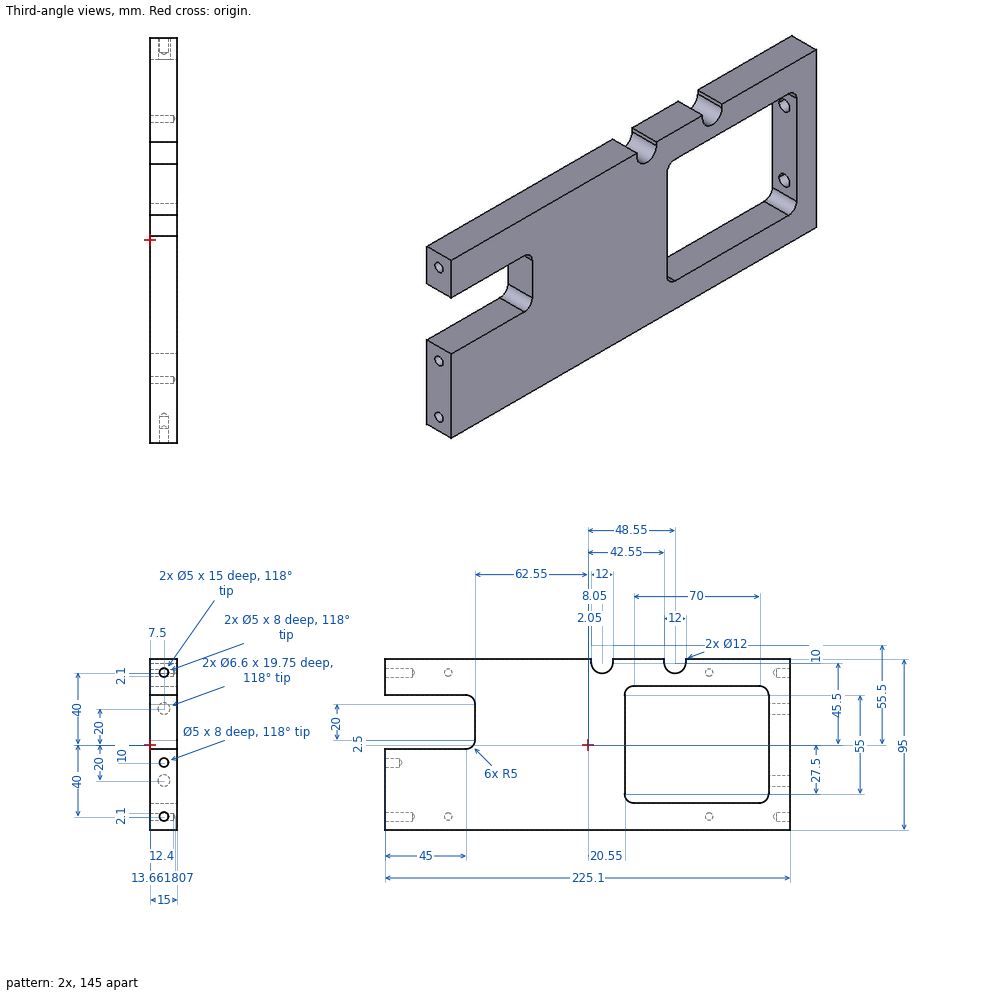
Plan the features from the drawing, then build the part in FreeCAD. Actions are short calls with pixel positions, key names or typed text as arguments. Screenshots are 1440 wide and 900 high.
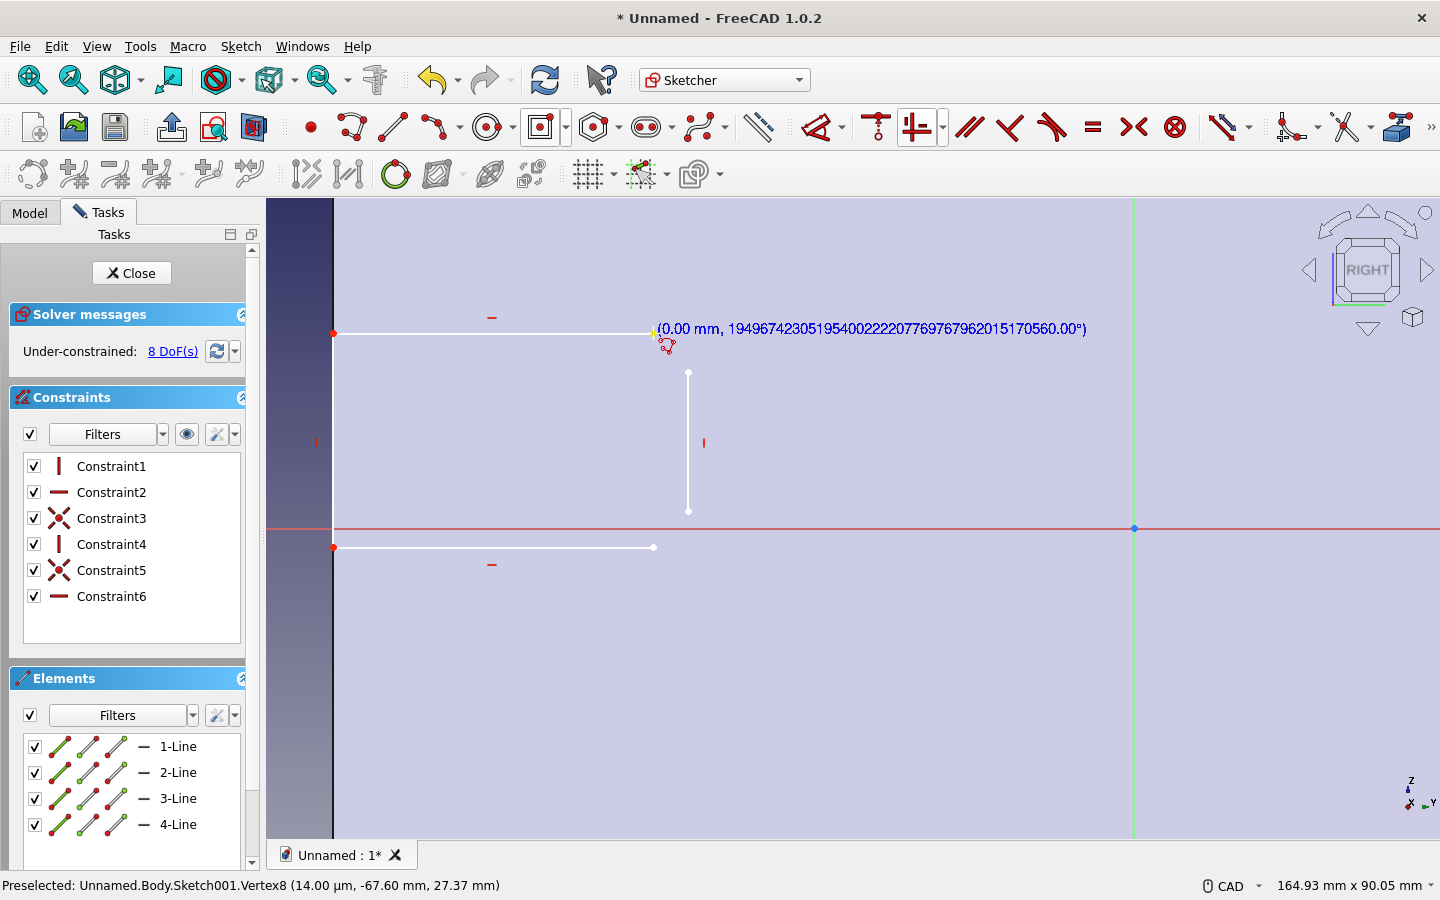
click(434, 128)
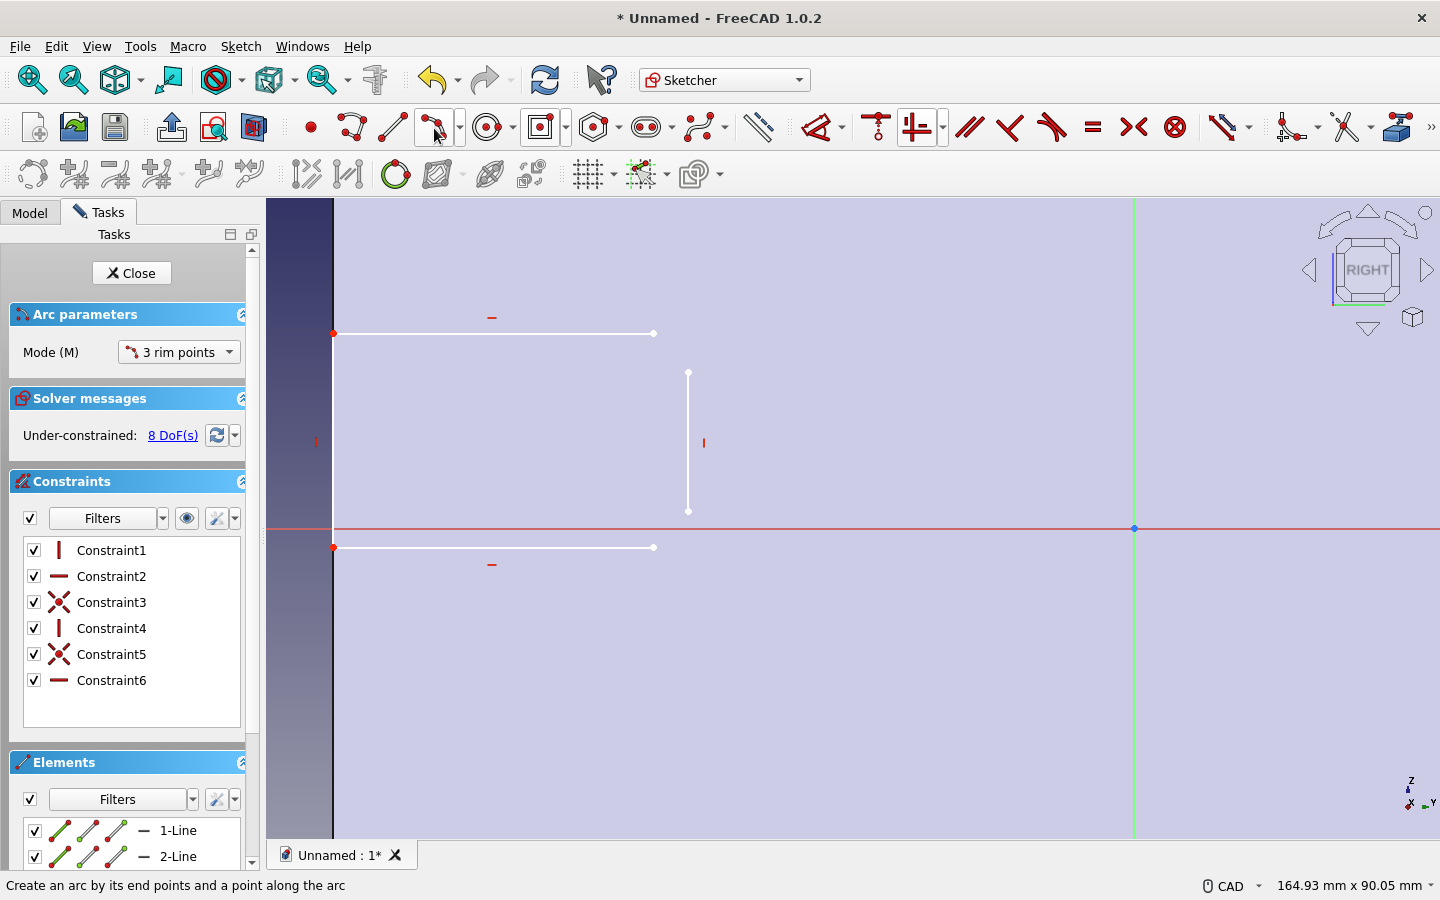
click(688, 512)
click(653, 548)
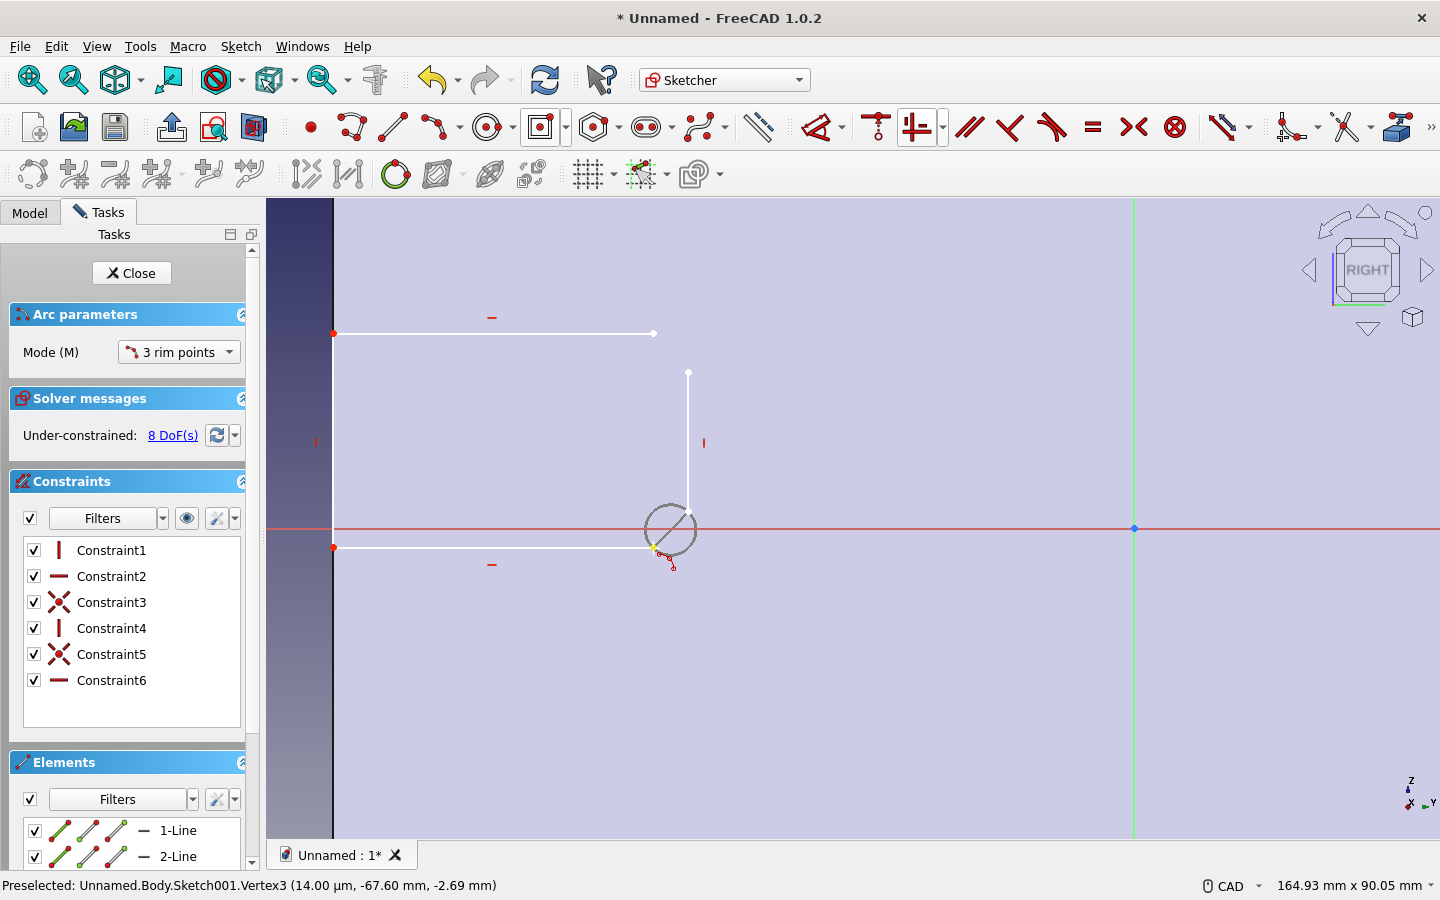
scroll(674, 540, up, 3)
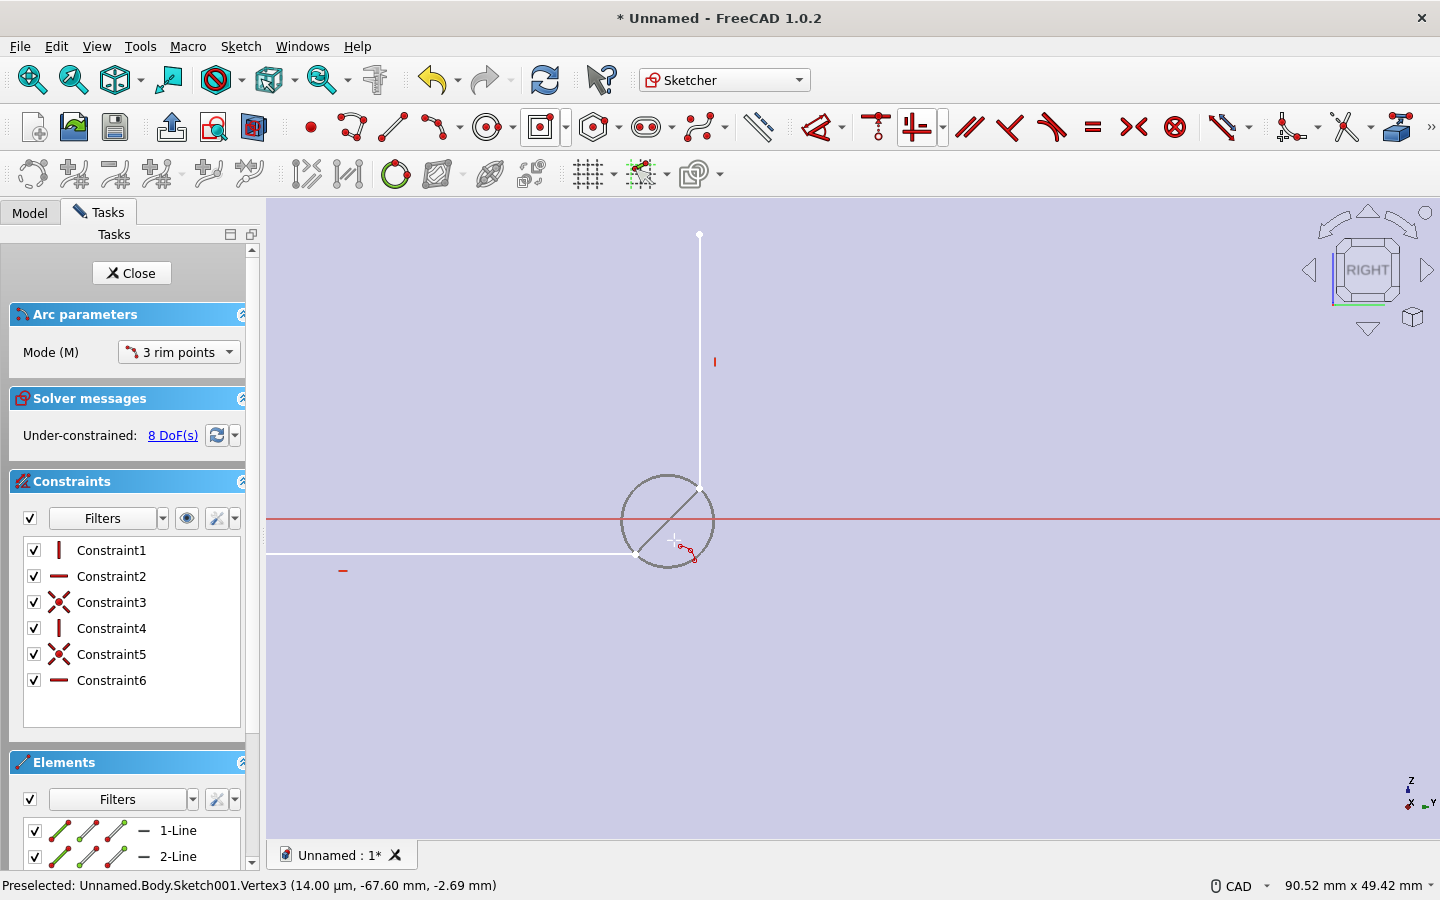
click(674, 539)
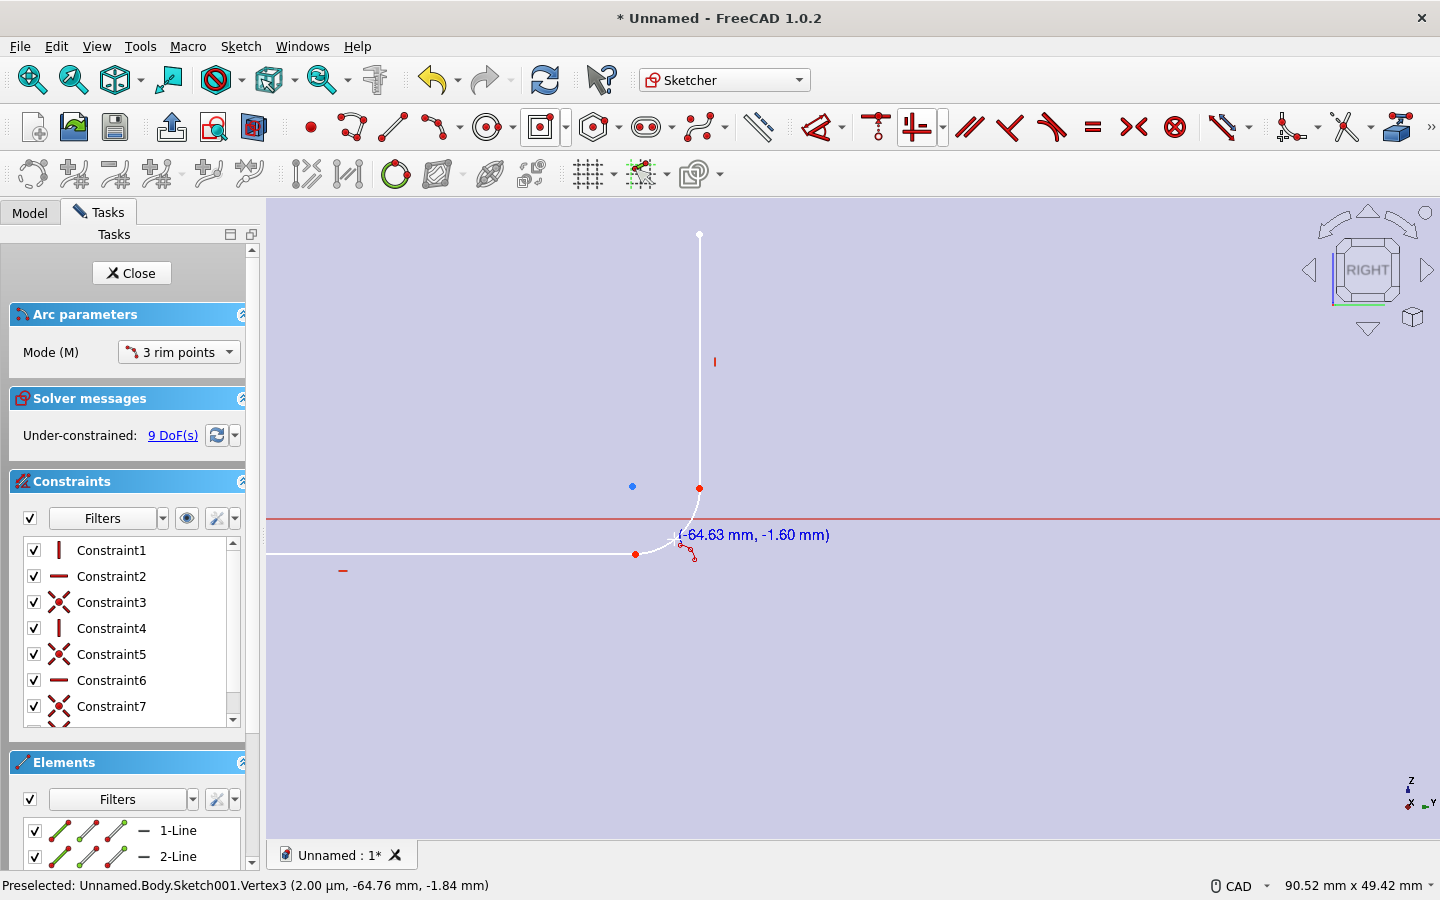
scroll(572, 518, down, 7)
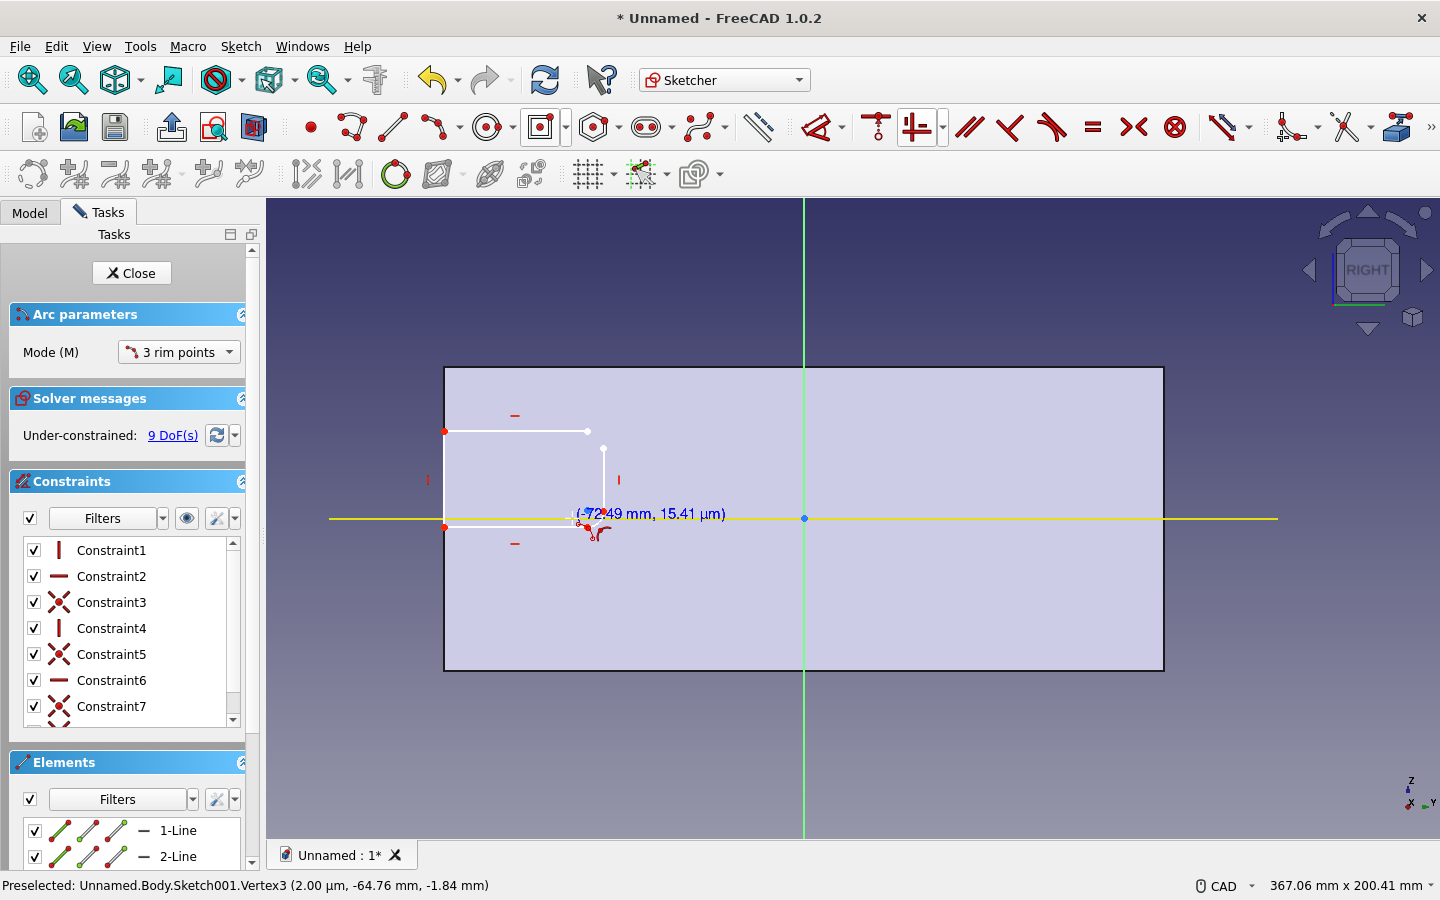
click(588, 431)
click(604, 448)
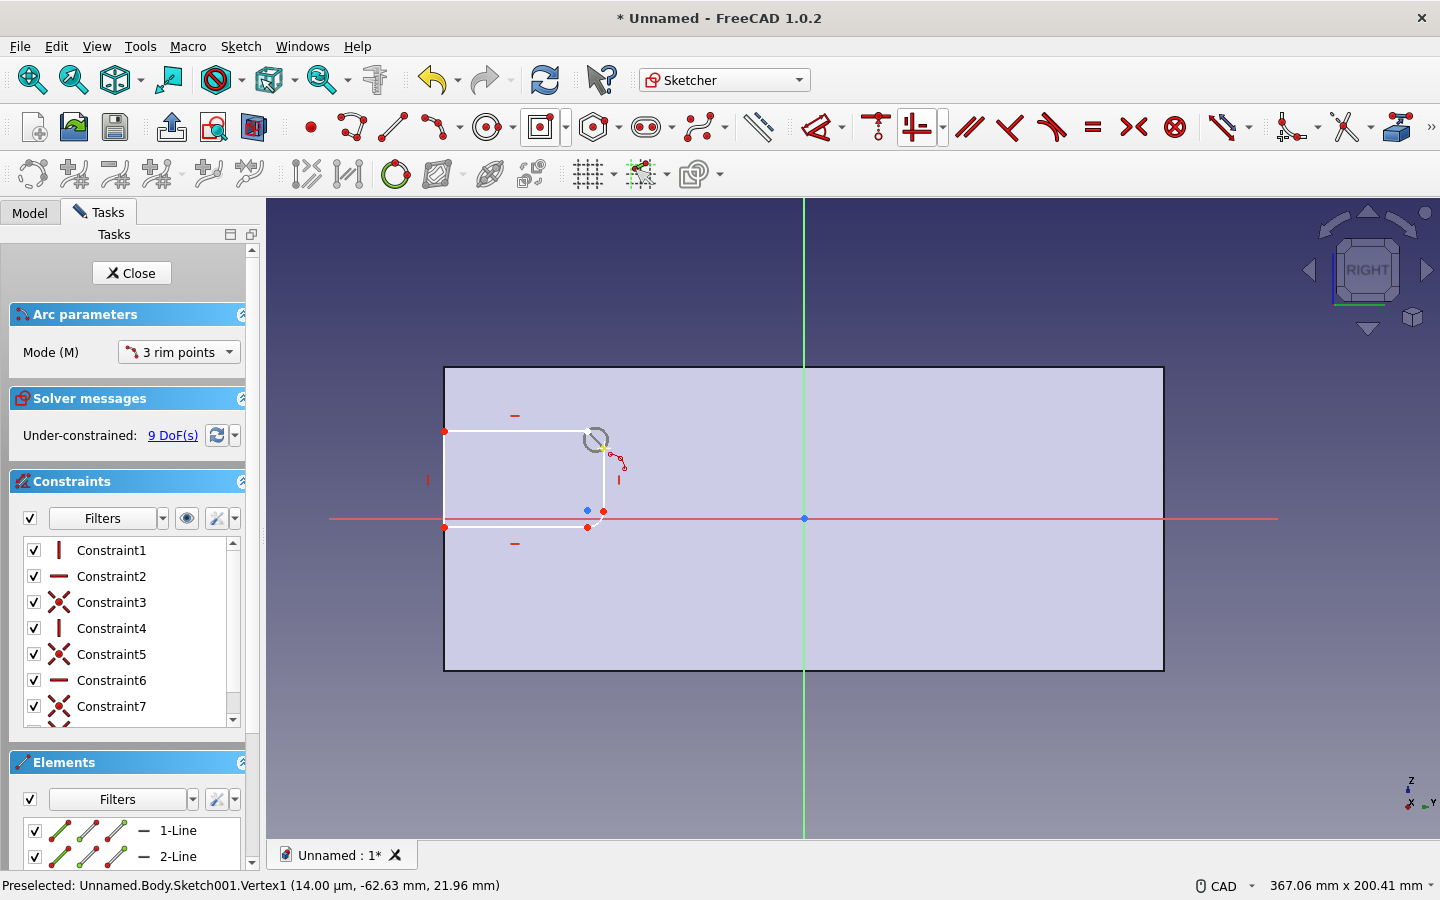
scroll(599, 435, up, 7)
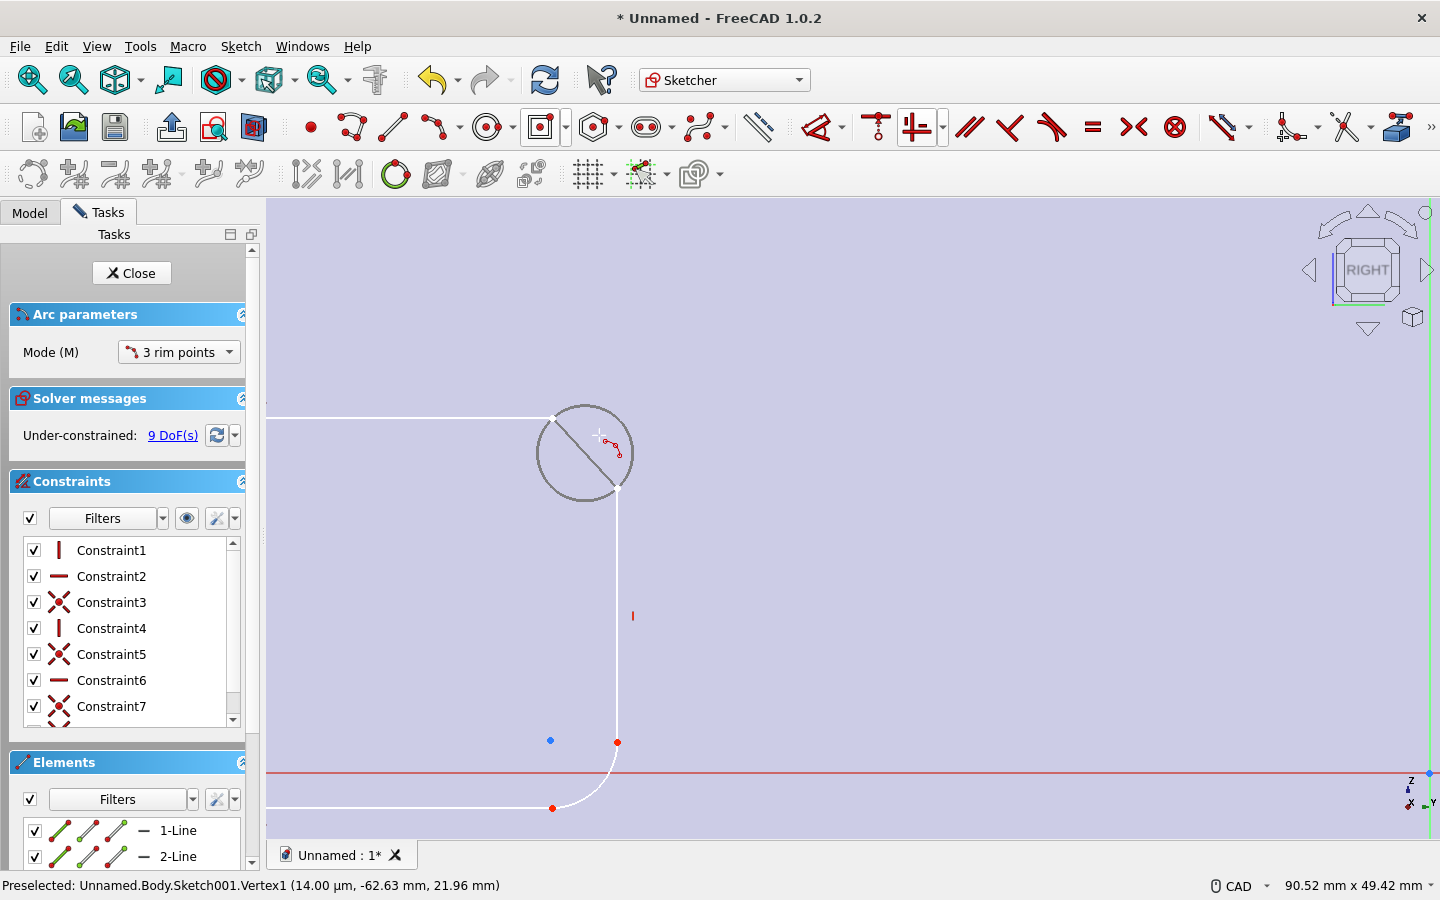
click(599, 435)